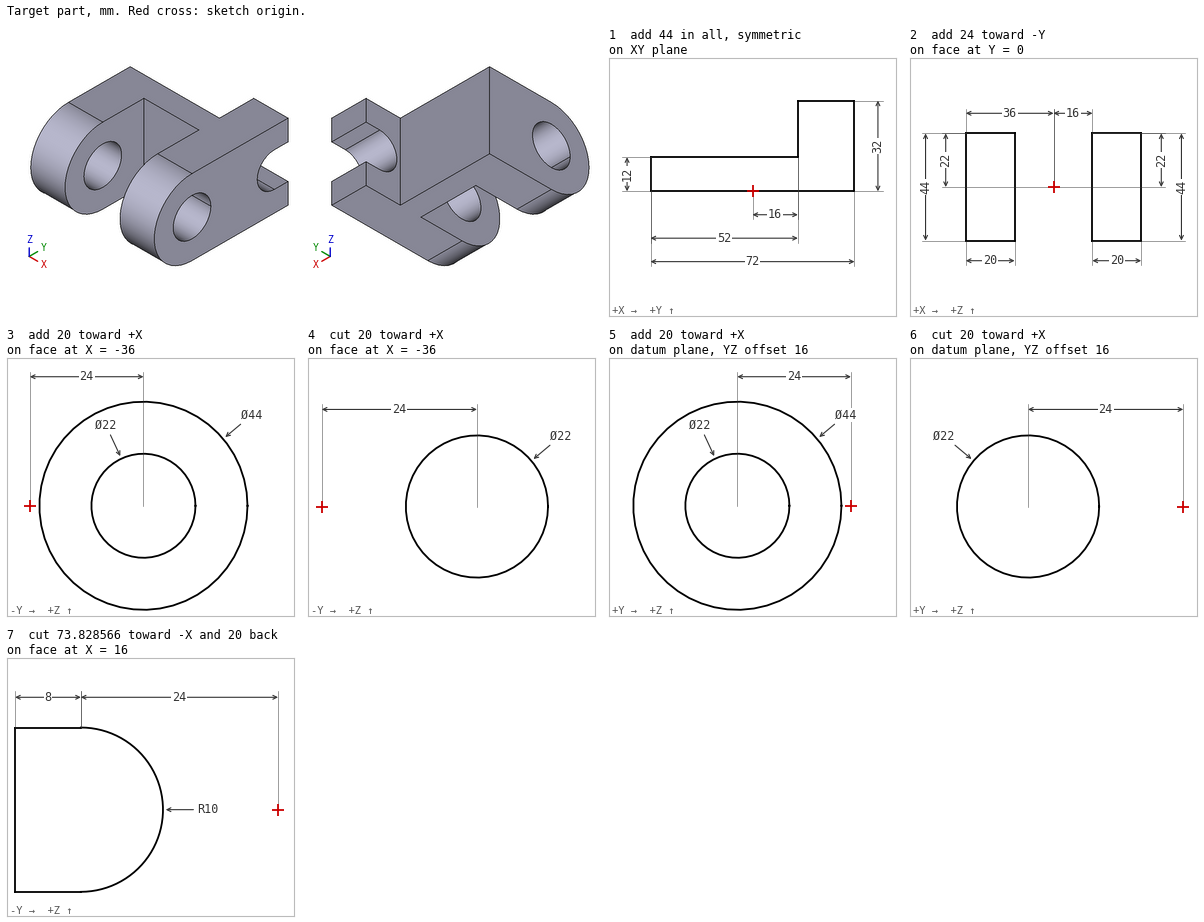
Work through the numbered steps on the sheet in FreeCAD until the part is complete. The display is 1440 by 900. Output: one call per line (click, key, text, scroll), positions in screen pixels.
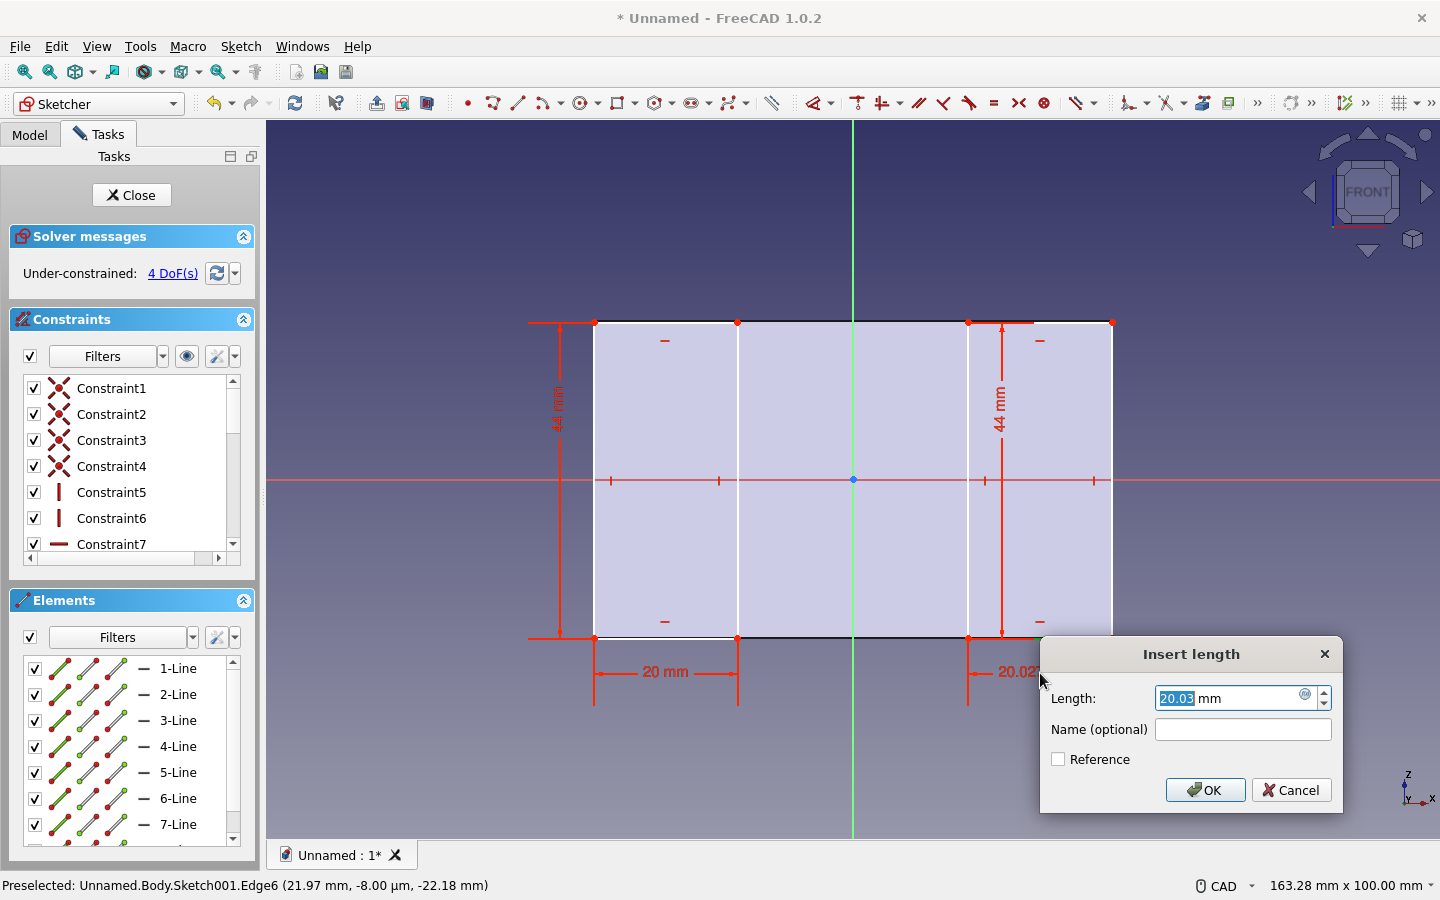
text(20)
key(Return)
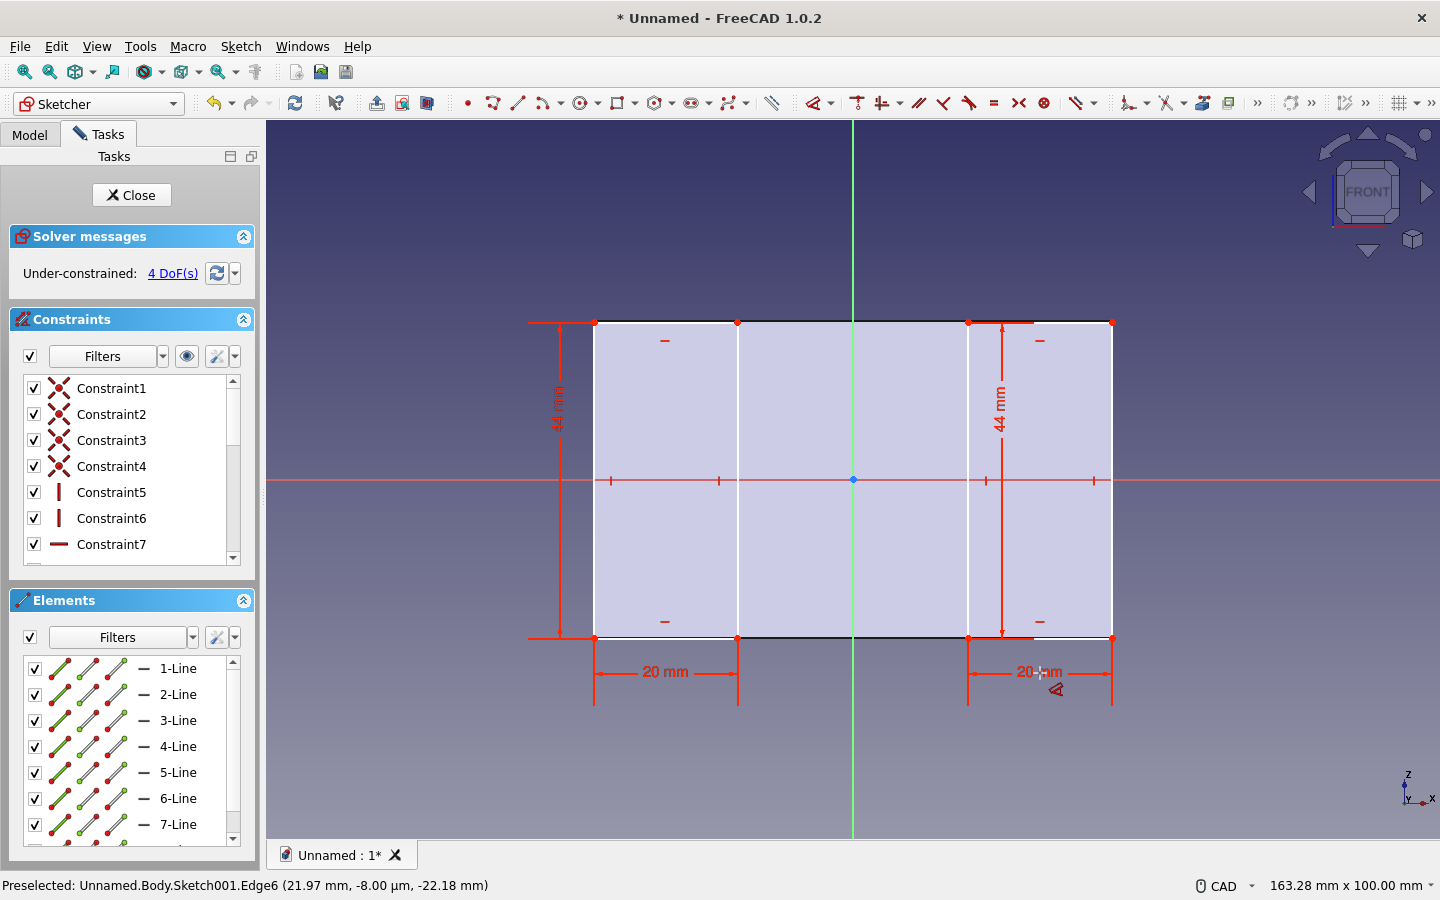
click(594, 323)
click(723, 289)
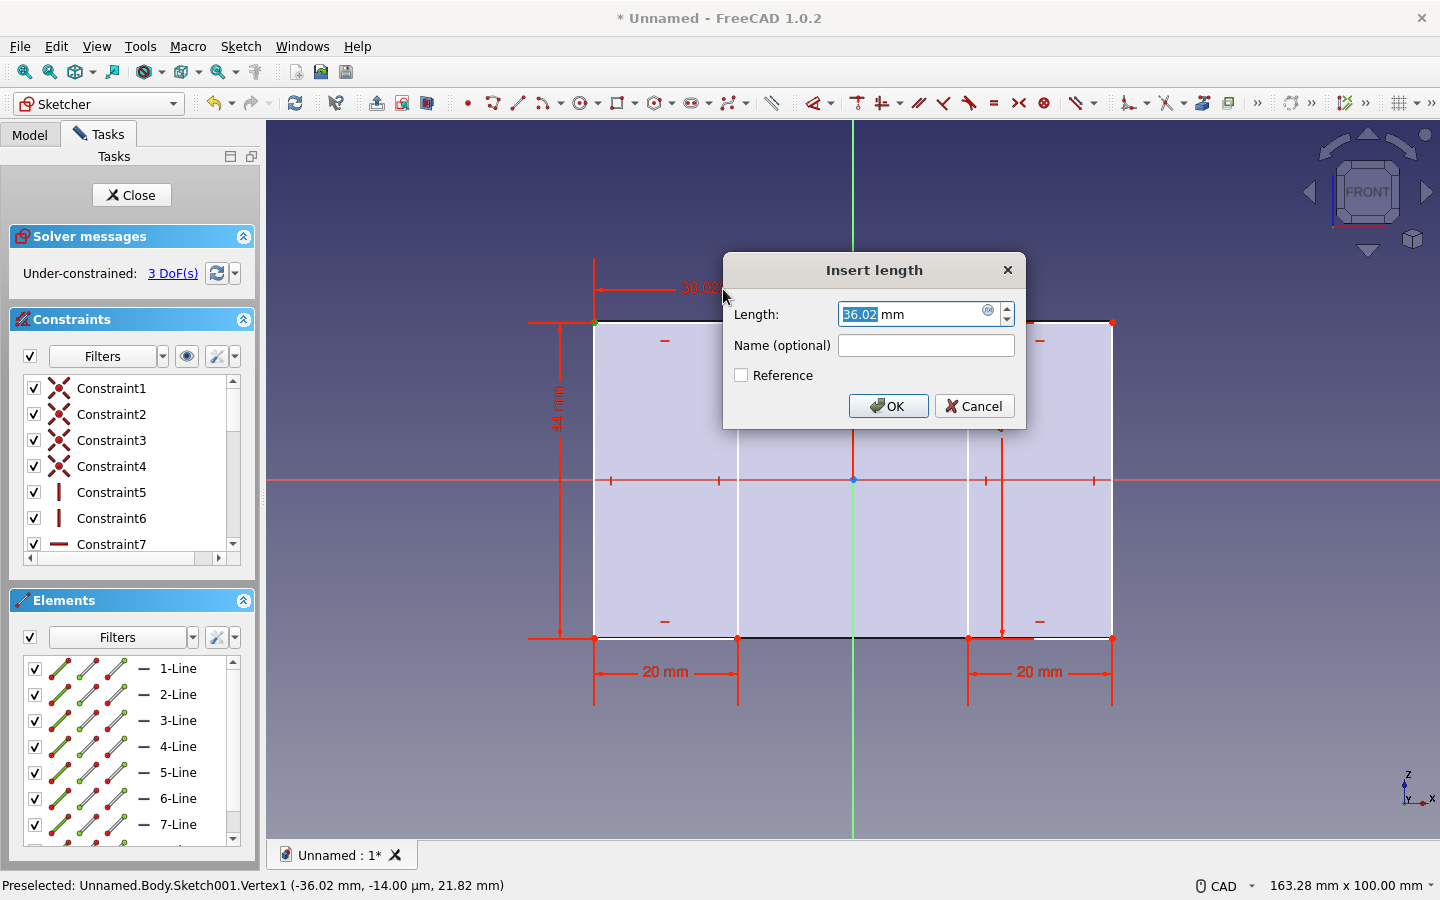
text(36)
key(Return)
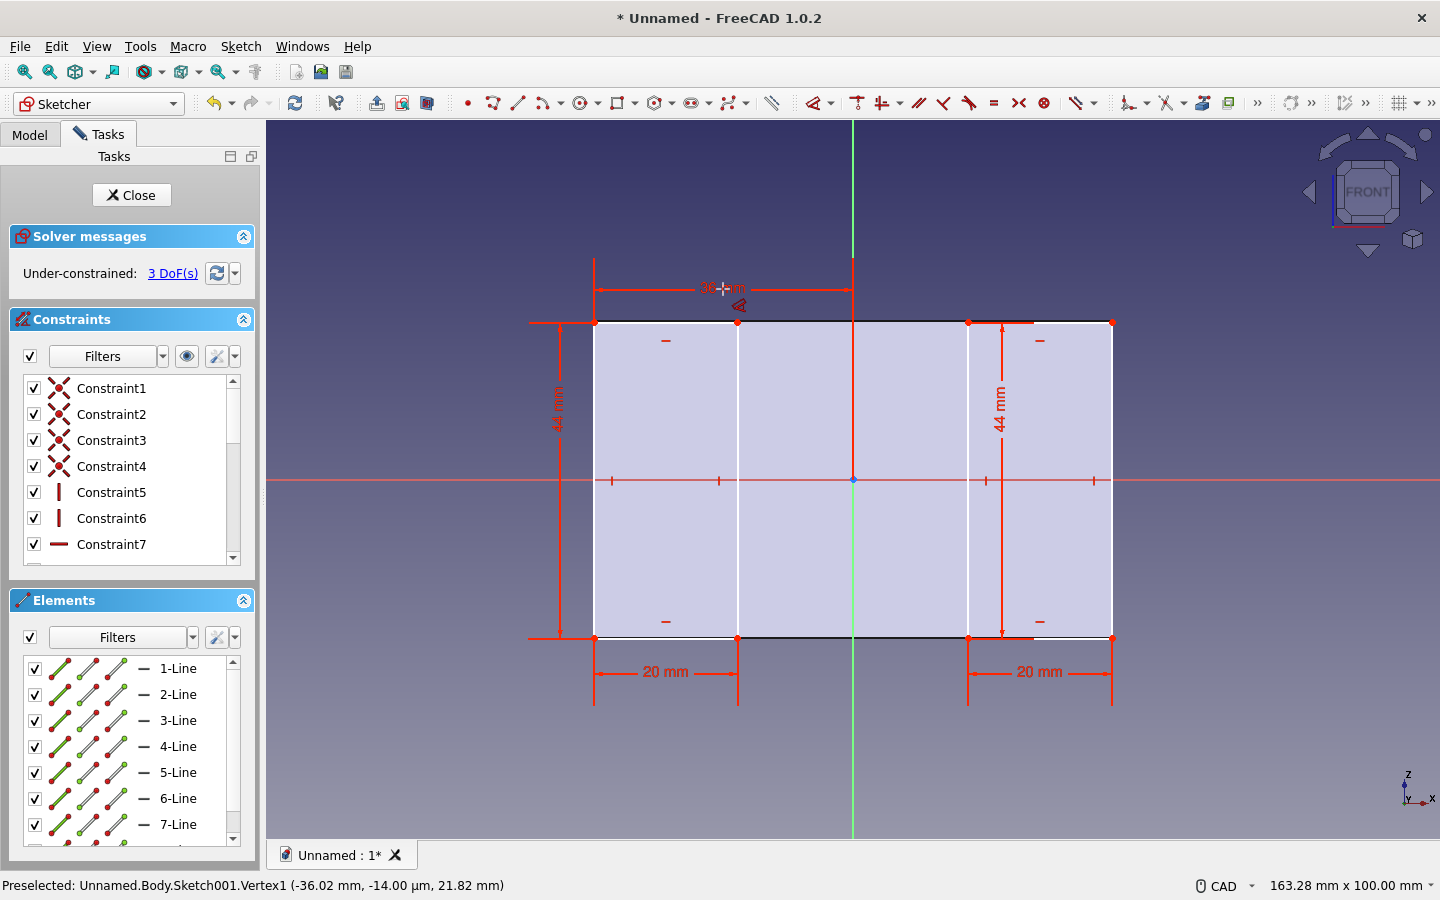
click(594, 323)
click(560, 365)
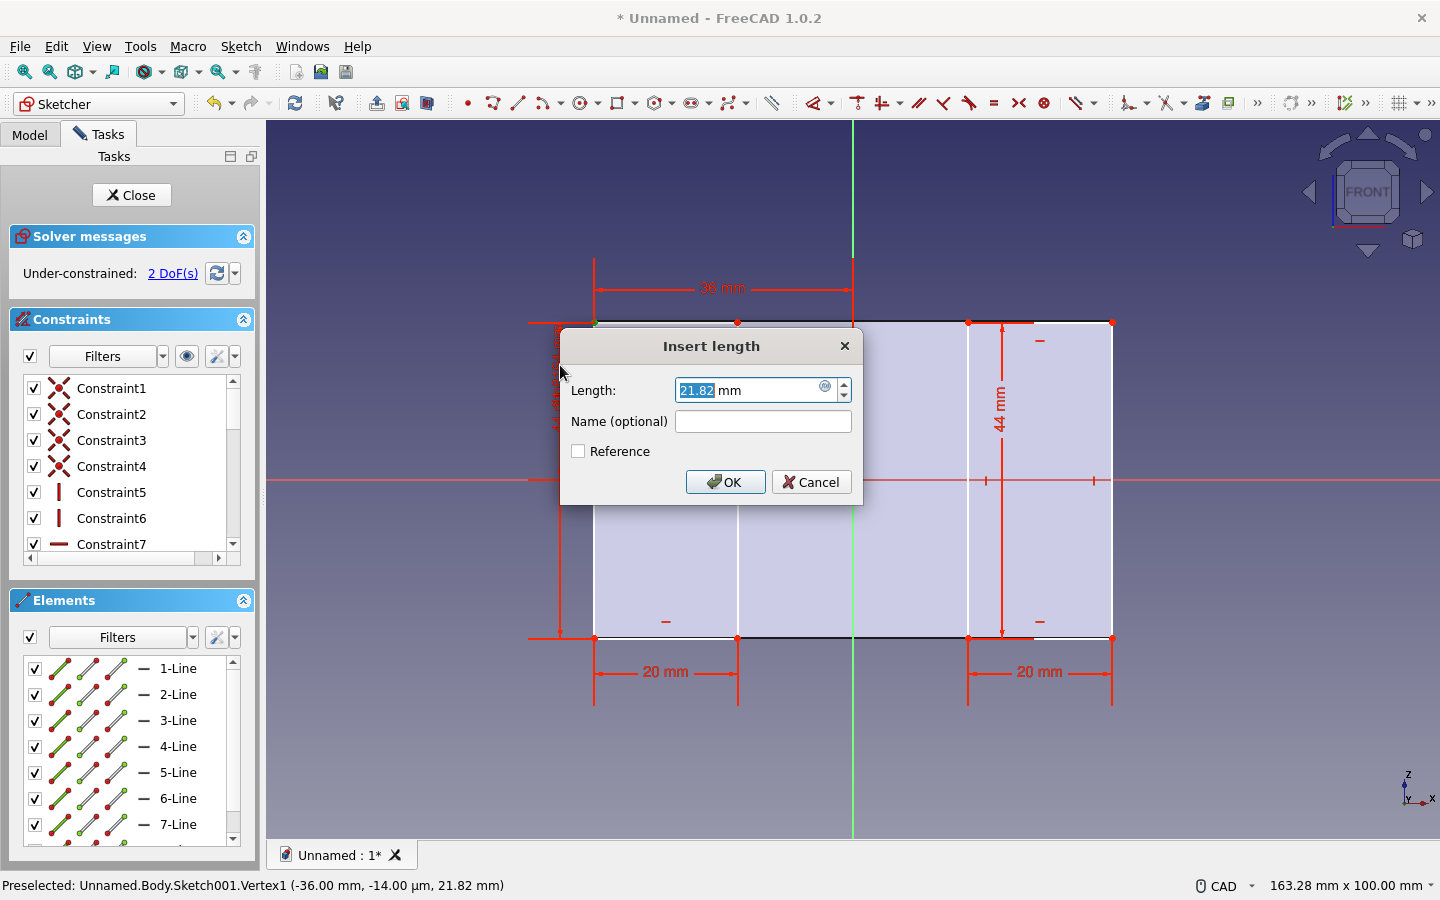
text(22)
key(Return)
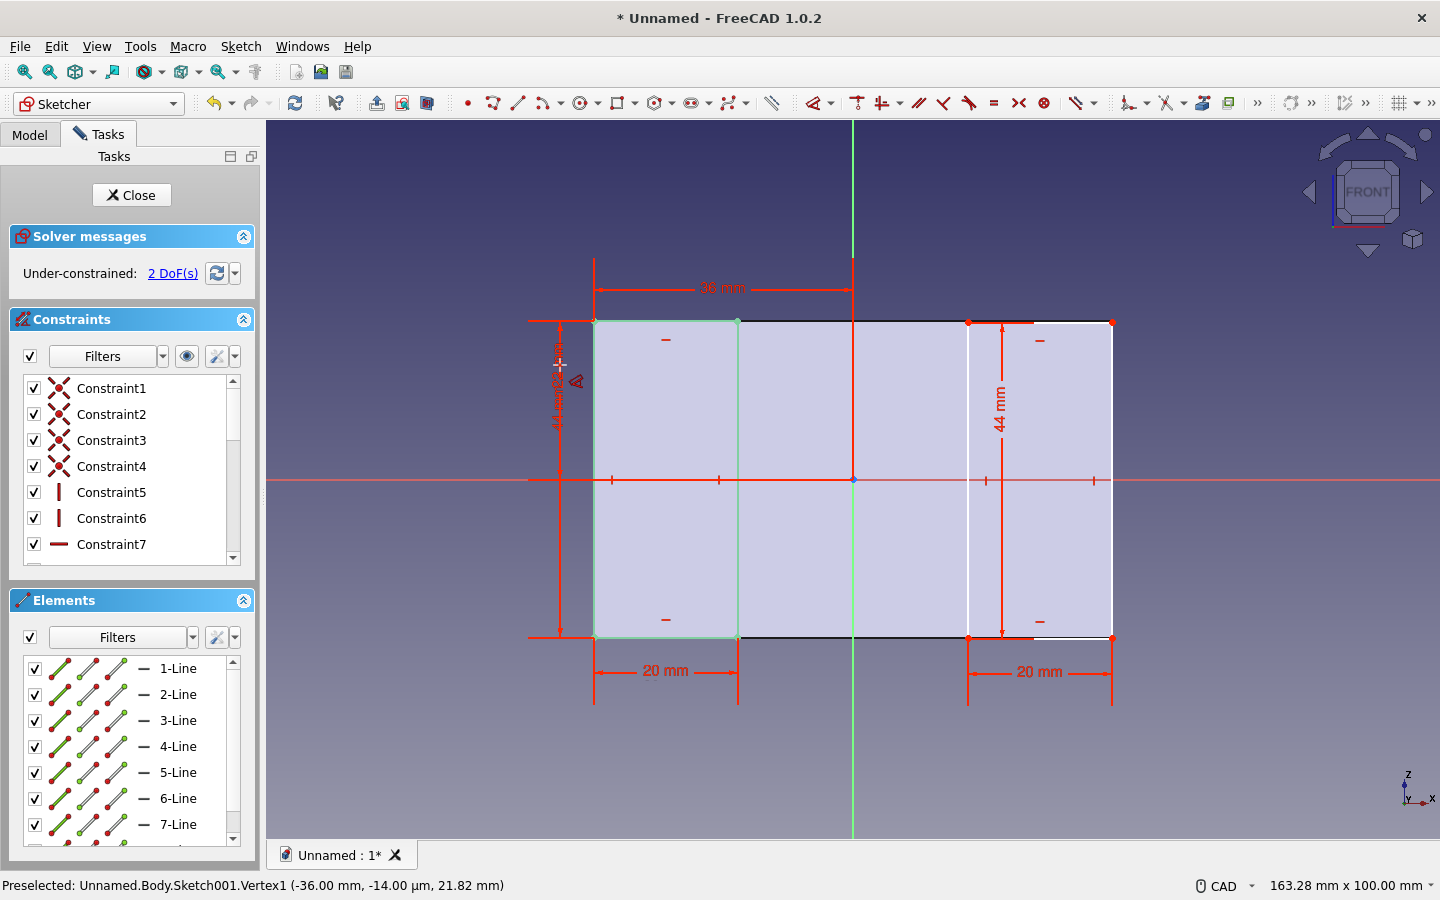
click(968, 323)
click(911, 289)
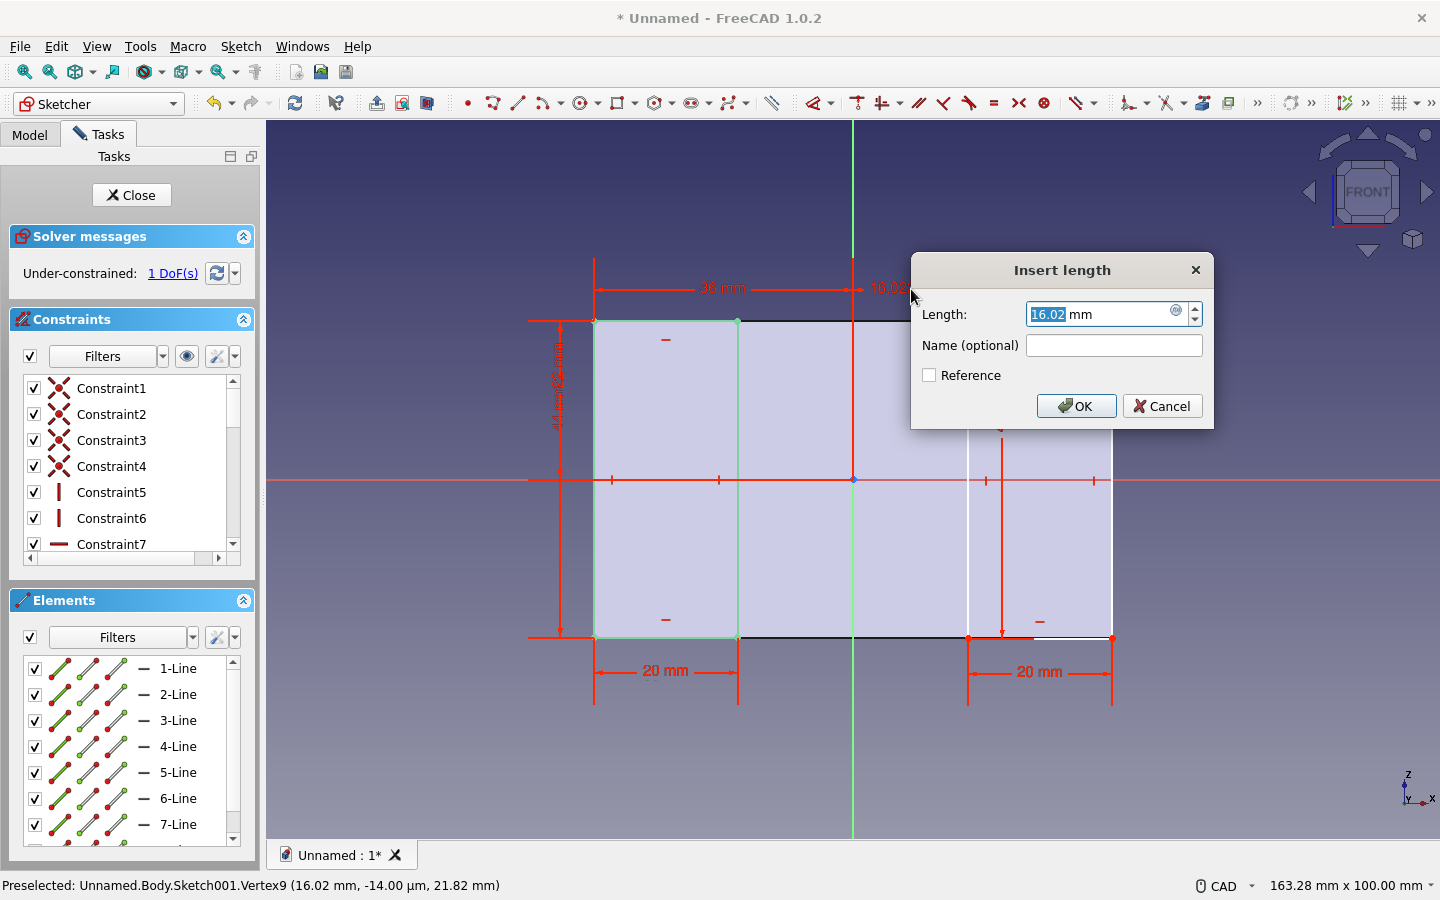
text(16)
key(Return)